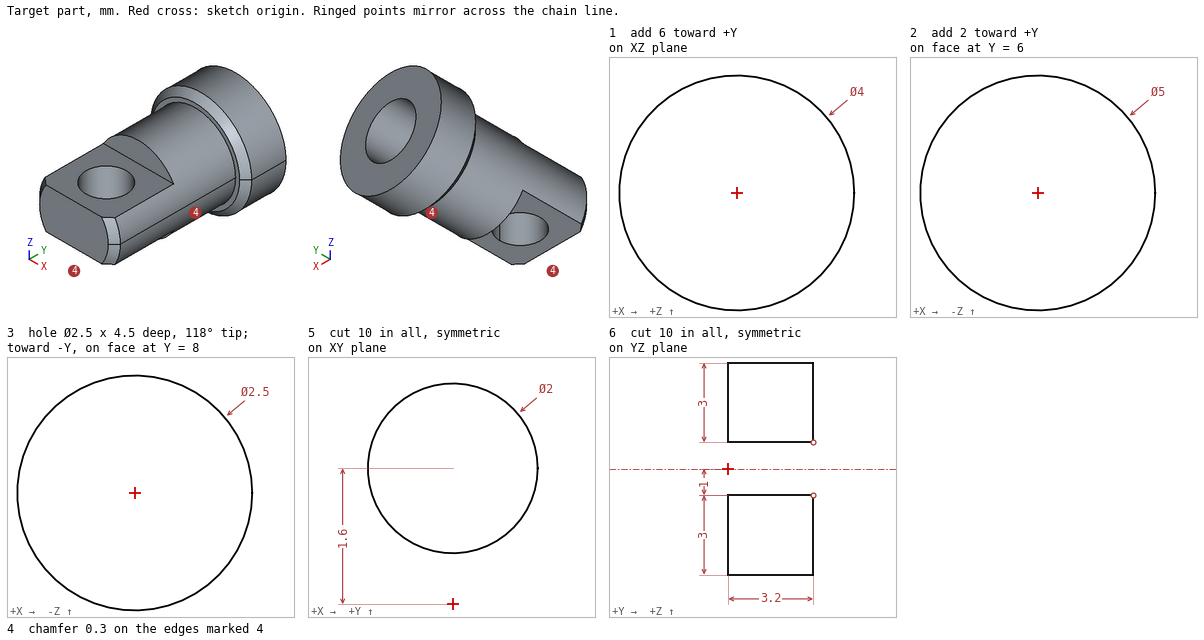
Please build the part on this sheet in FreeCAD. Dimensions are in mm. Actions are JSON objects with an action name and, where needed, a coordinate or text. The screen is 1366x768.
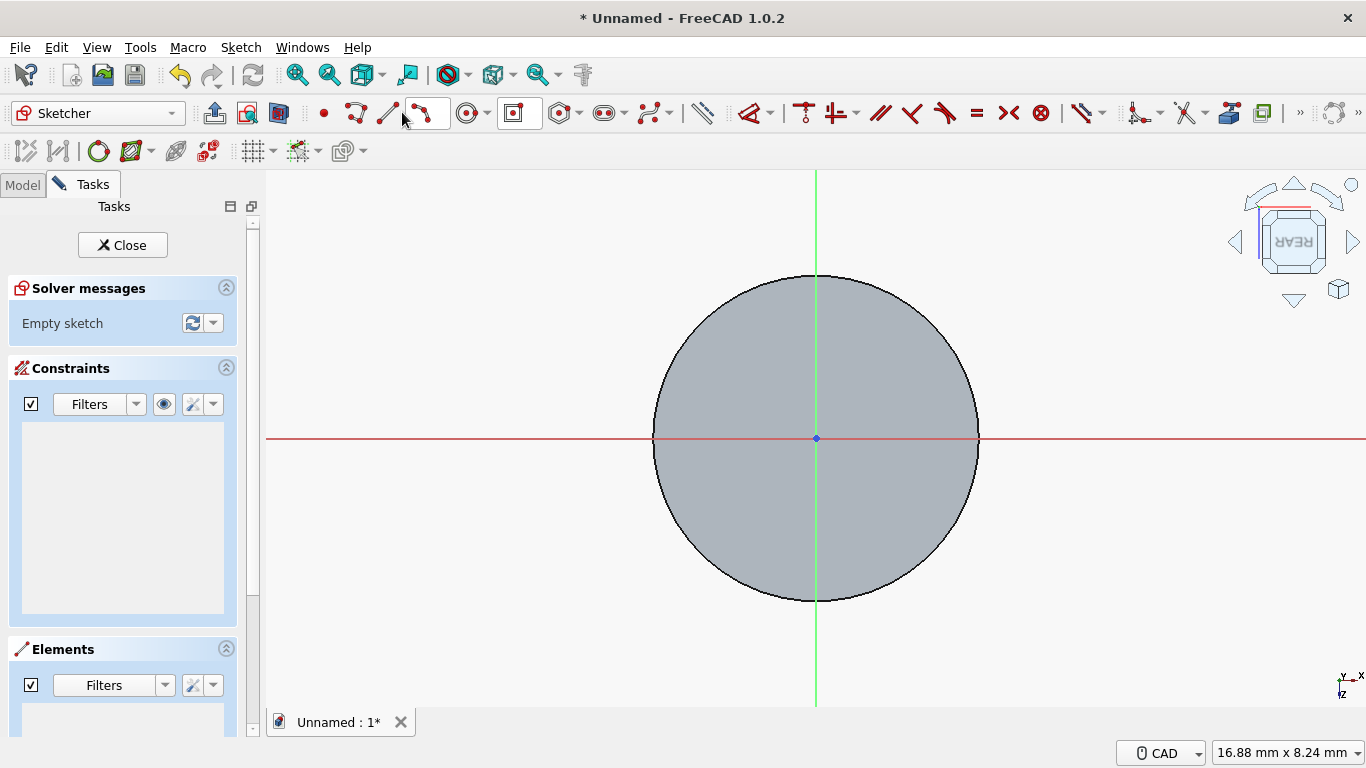
{"action": "scroll", "coordinate": [872, 439], "scroll_direction": "up", "scroll_amount": 4}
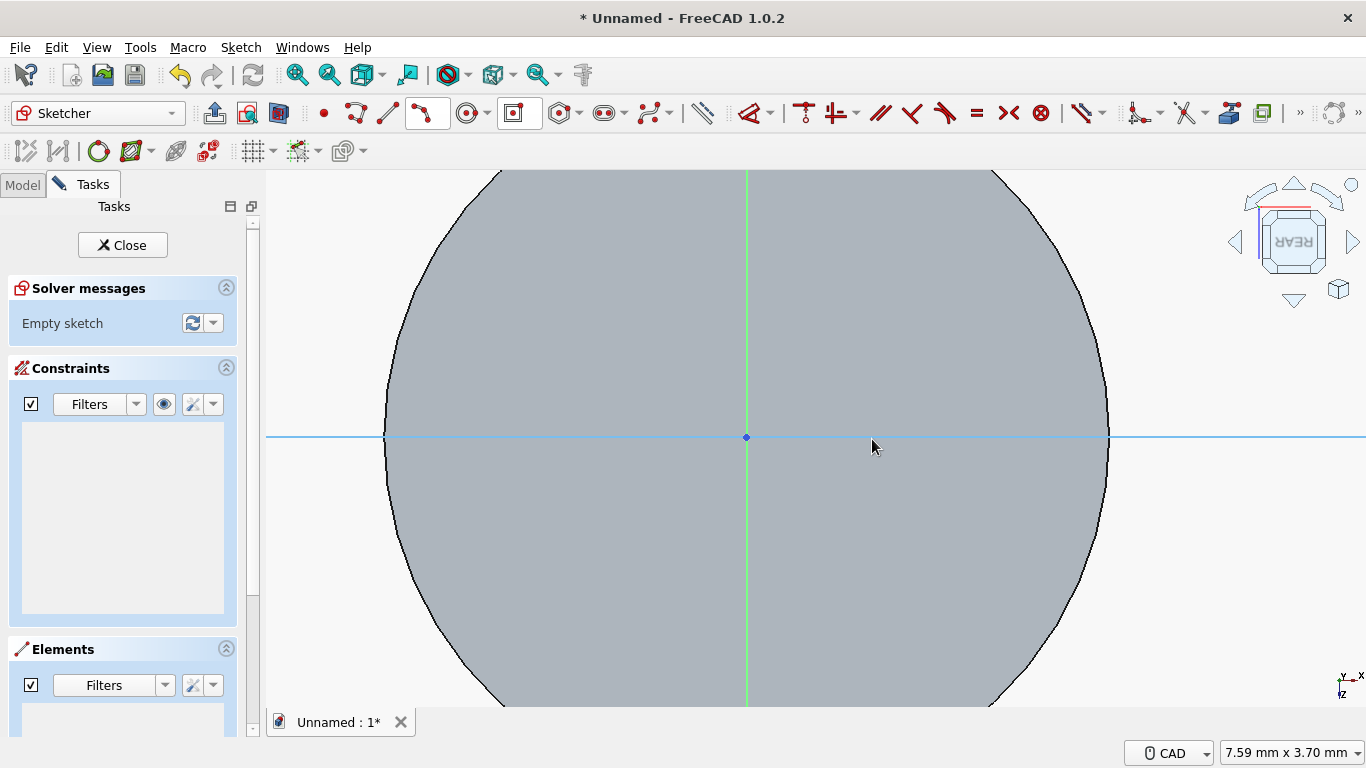
{"action": "key", "text": "g c"}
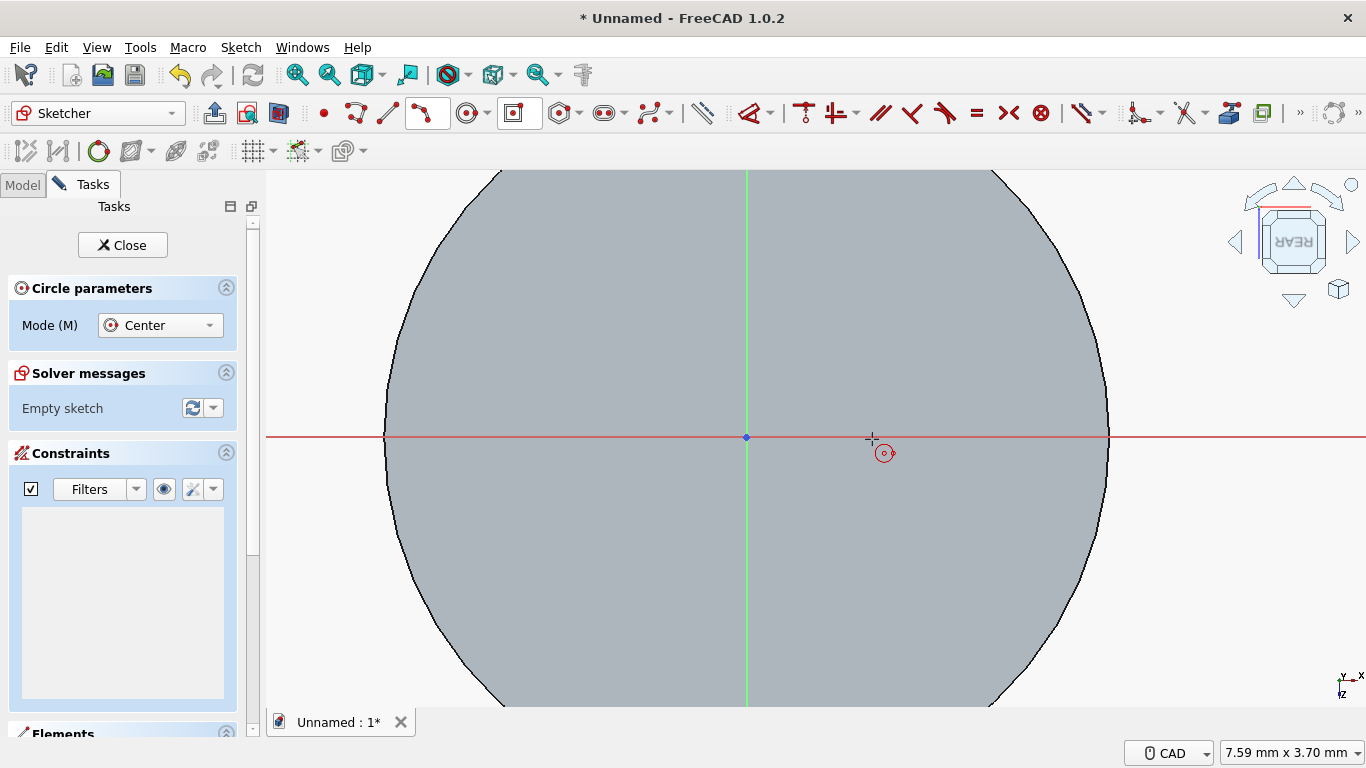
{"action": "left_click", "coordinate": [747, 437]}
{"action": "left_click", "coordinate": [875, 309]}
{"action": "key", "text": "Escape"}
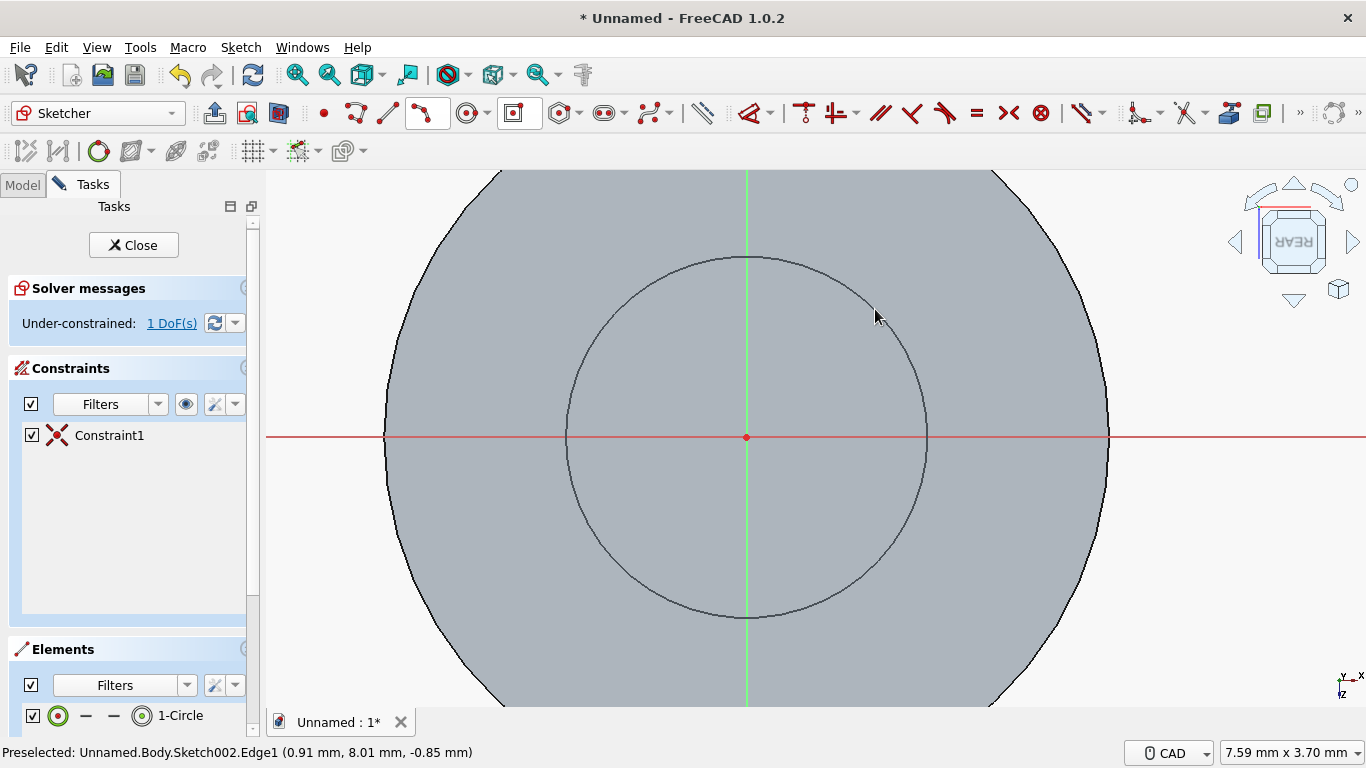
{"action": "left_click", "coordinate": [874, 309]}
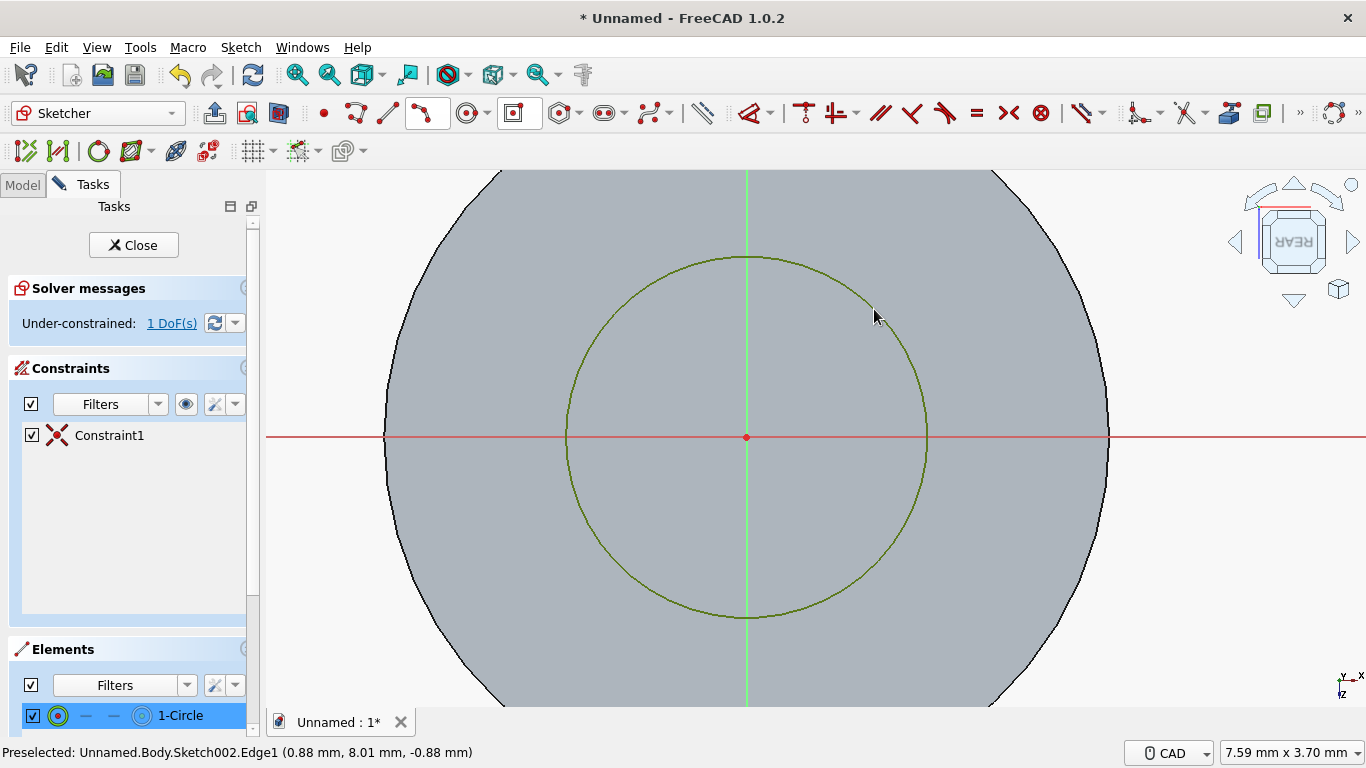
{"action": "left_click", "coordinate": [772, 114]}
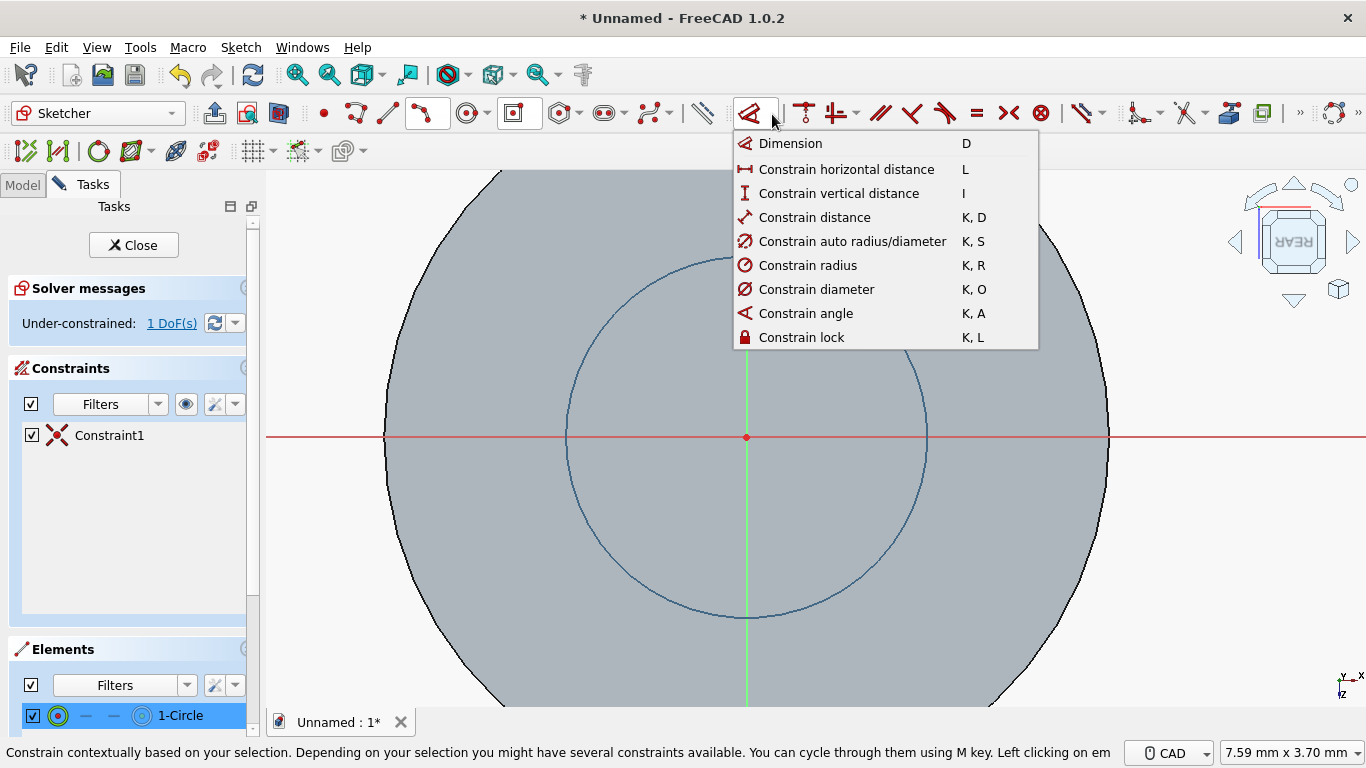
{"action": "left_click", "coordinate": [886, 289]}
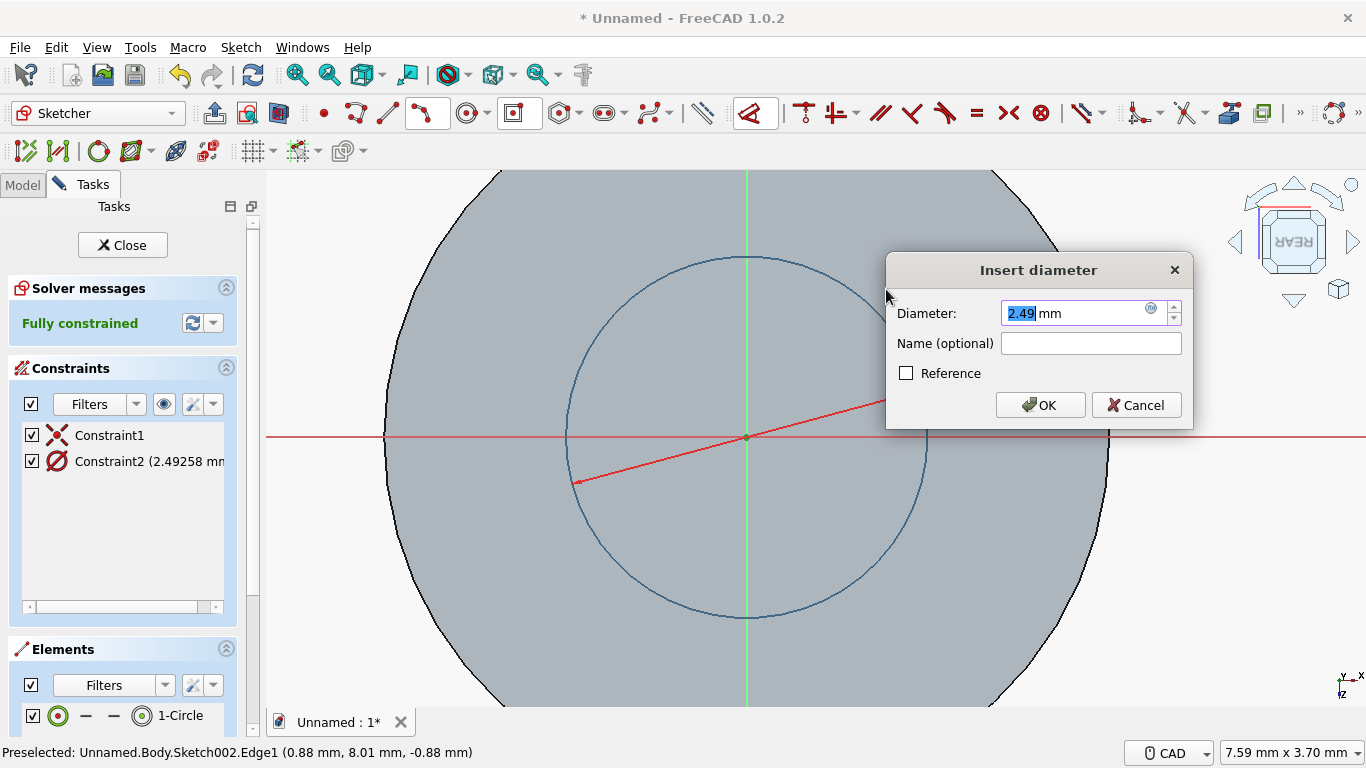
{"action": "type", "text": "2.5"}
{"action": "key", "text": "Return"}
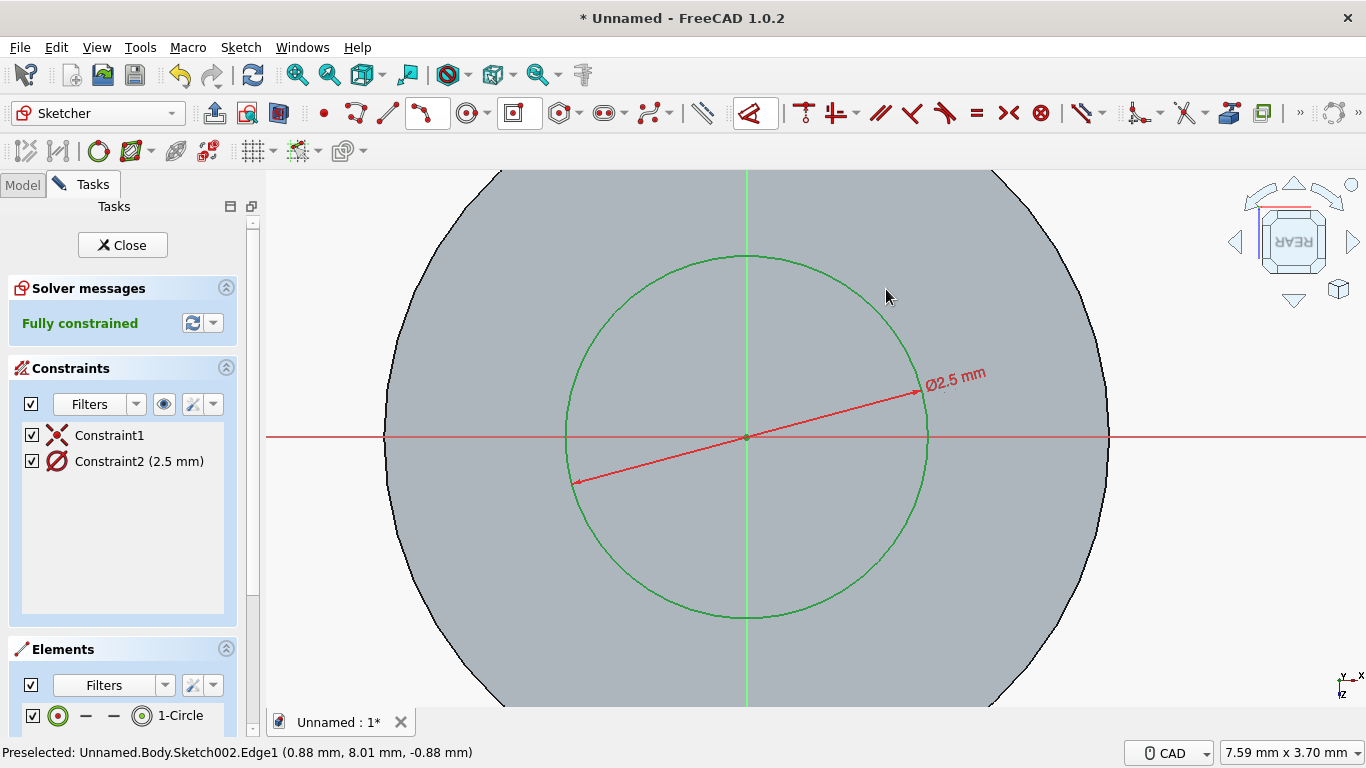
{"action": "left_click", "coordinate": [123, 245]}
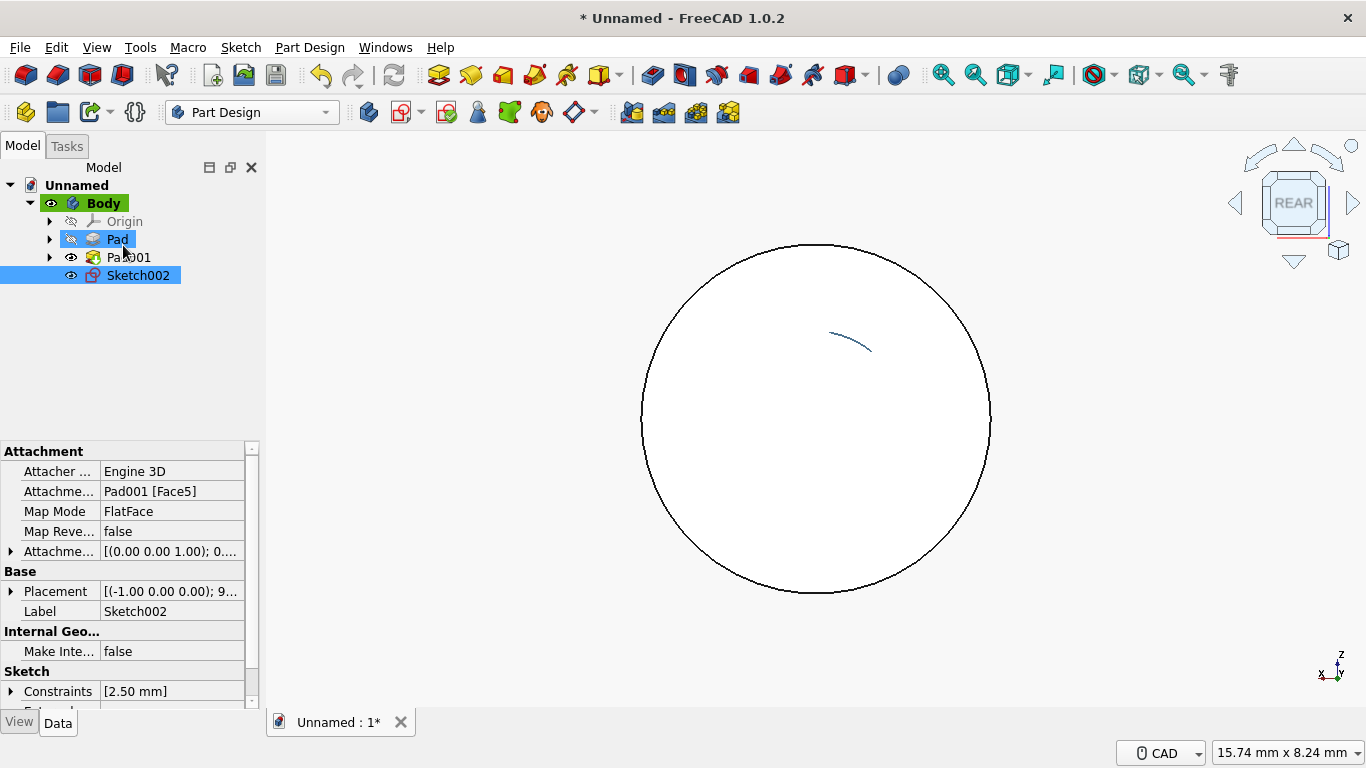
{"action": "left_click", "coordinate": [686, 76]}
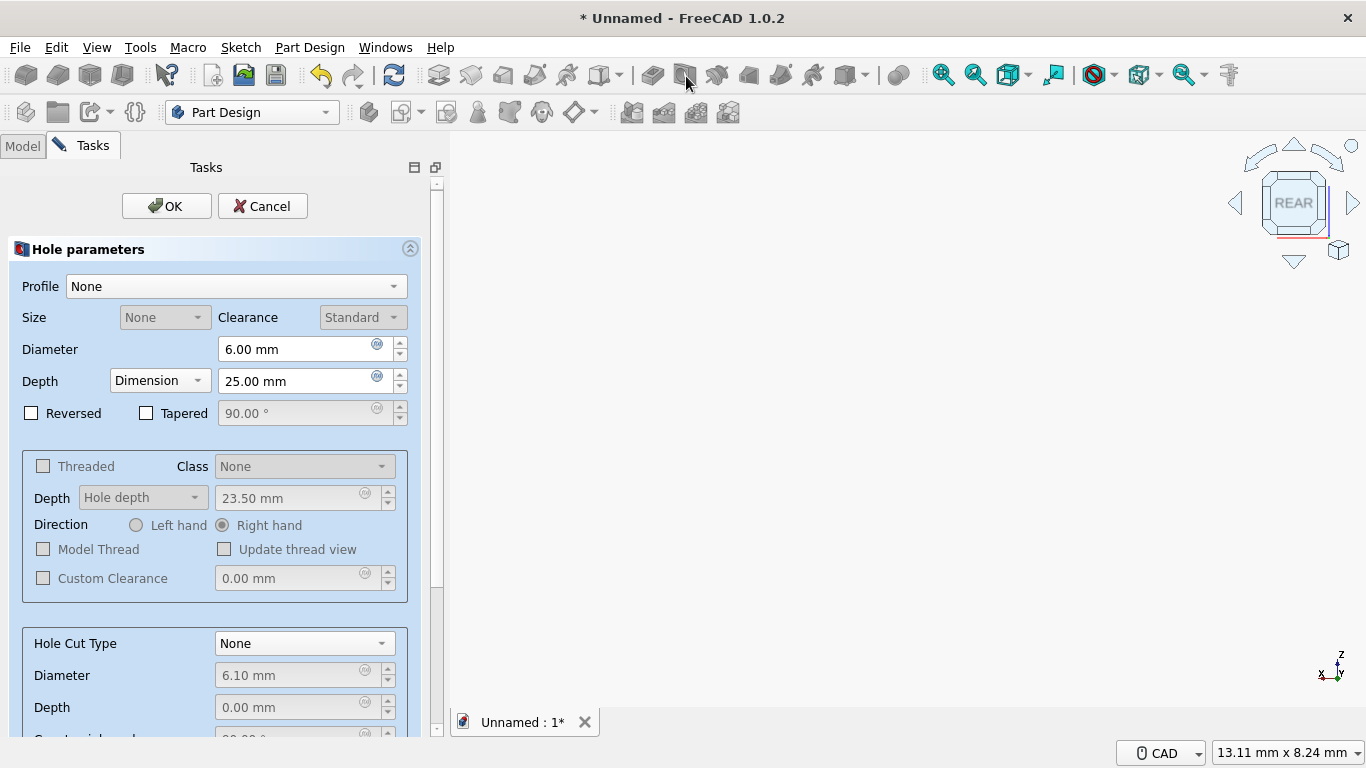
{"action": "triple_click", "coordinate": [305, 349]}